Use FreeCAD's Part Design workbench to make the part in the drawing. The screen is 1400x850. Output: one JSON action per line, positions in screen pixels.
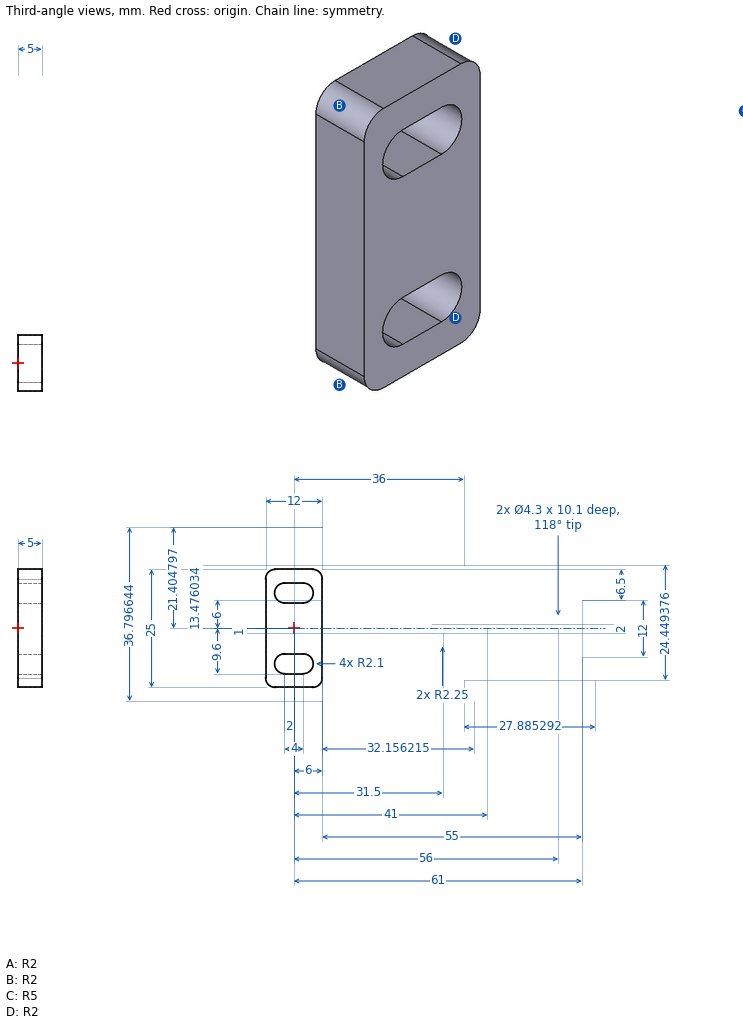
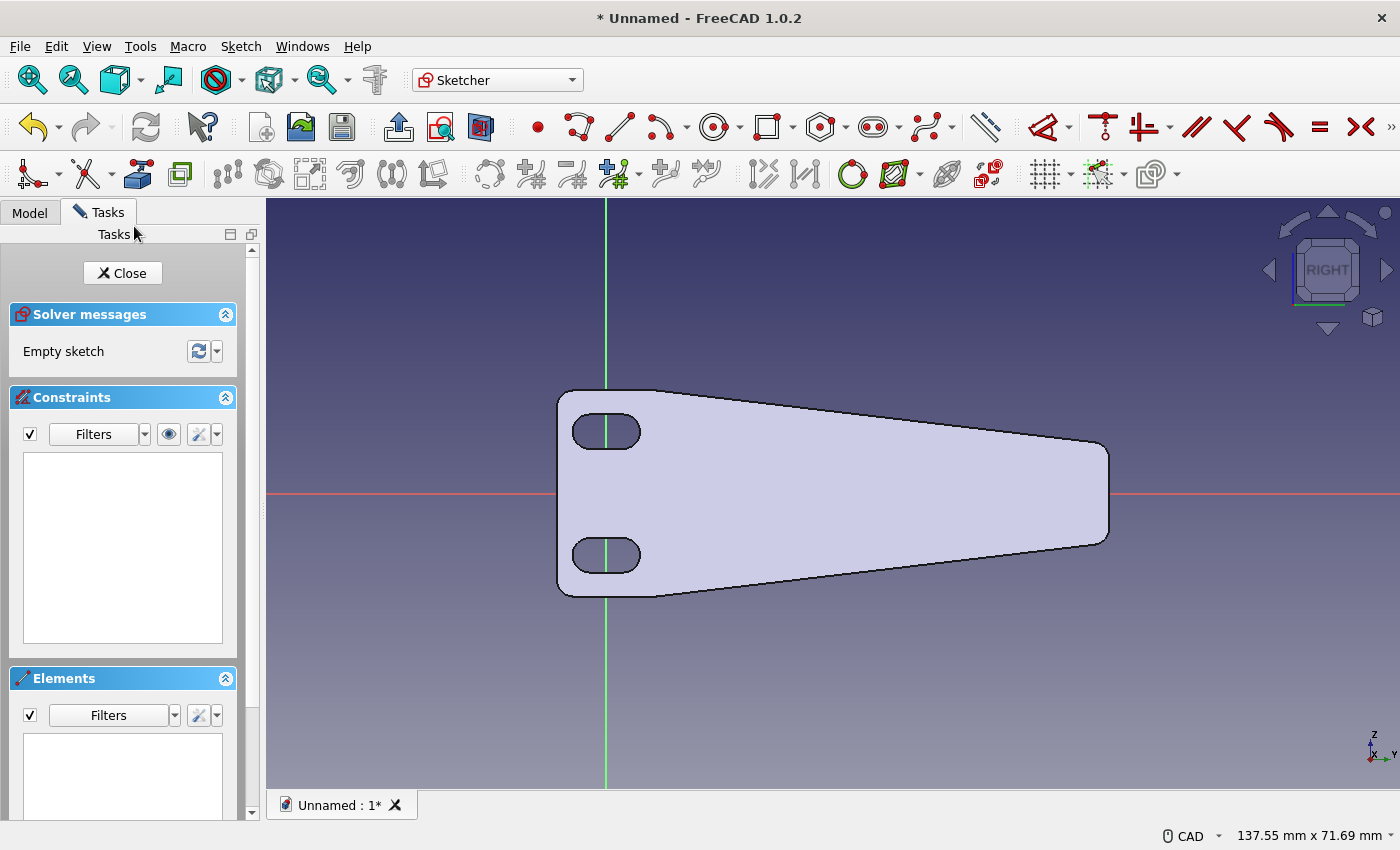
{"action": "left_click", "coordinate": [481, 128]}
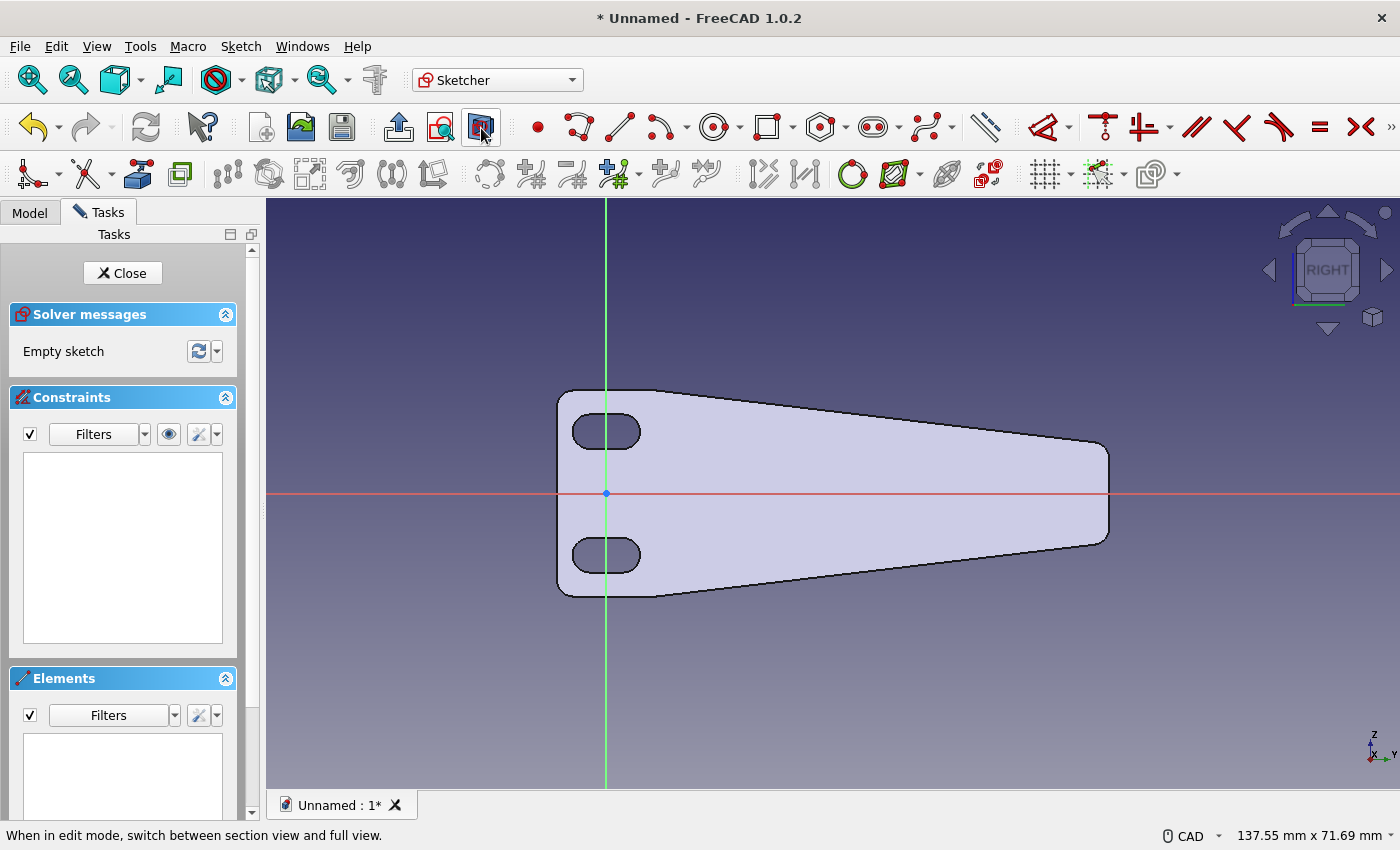
{"action": "scroll", "coordinate": [1085, 494], "scroll_direction": "up", "scroll_amount": 7}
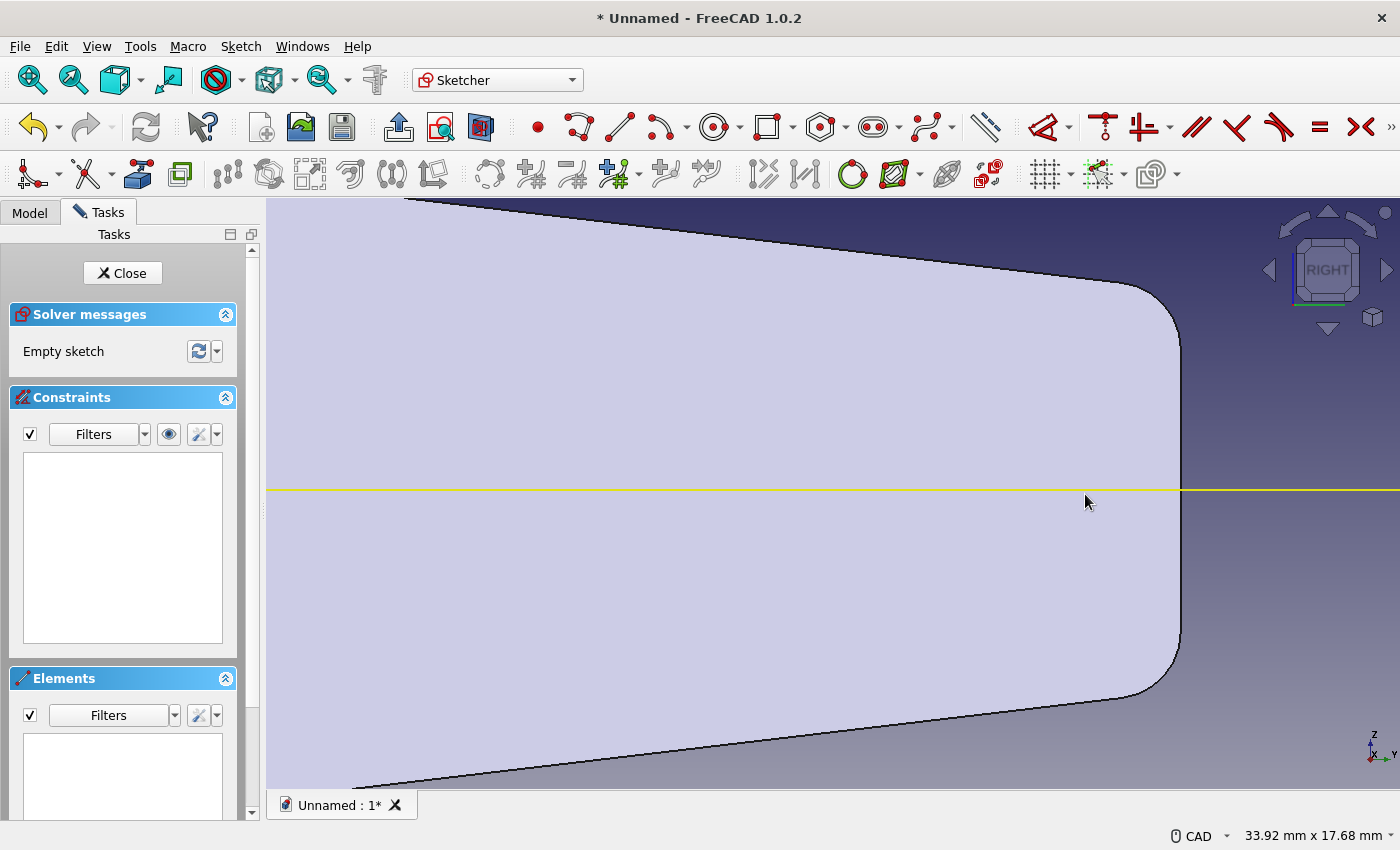
{"action": "left_click", "coordinate": [714, 128]}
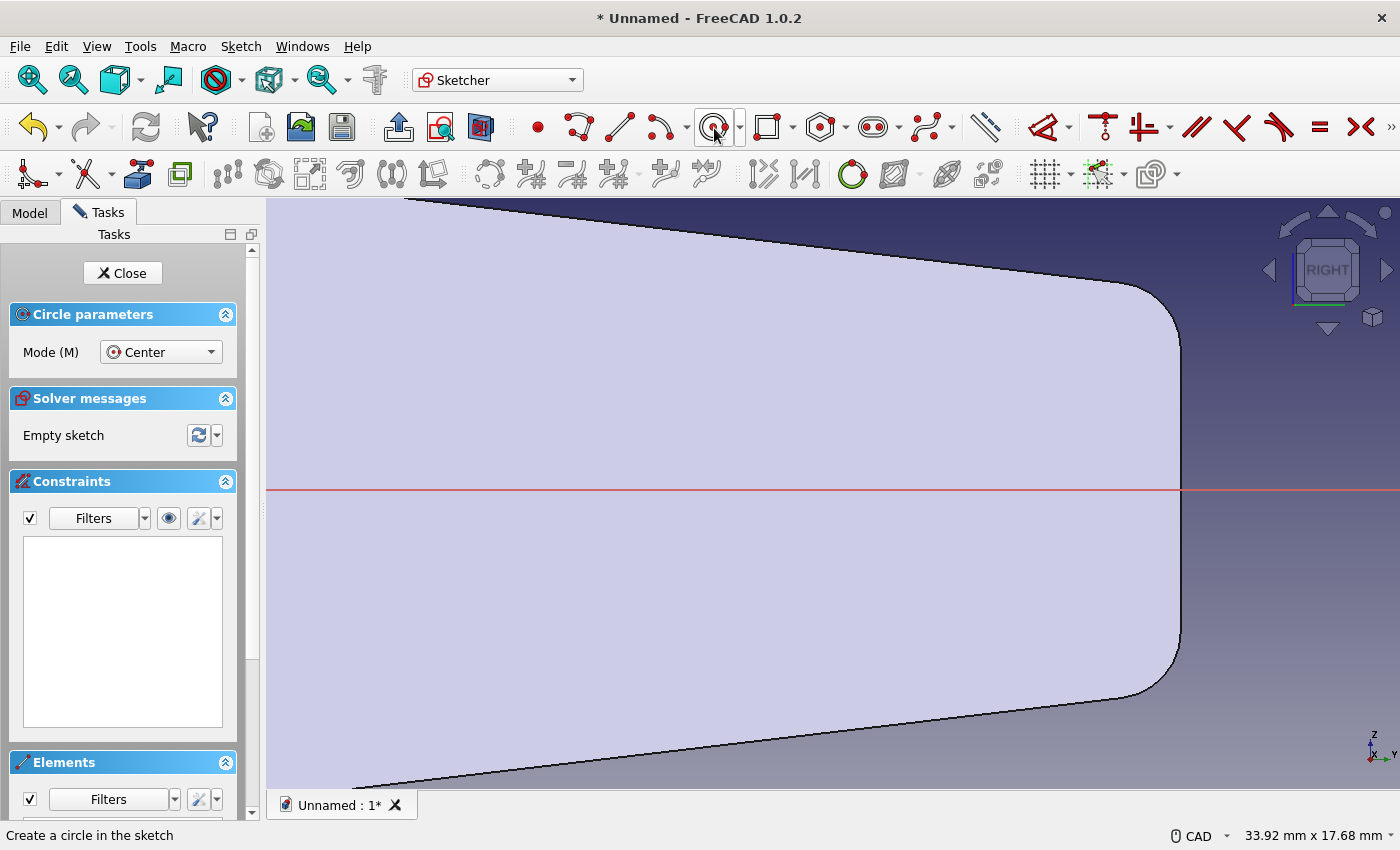
{"action": "left_click", "coordinate": [1014, 490]}
{"action": "left_click", "coordinate": [1065, 440]}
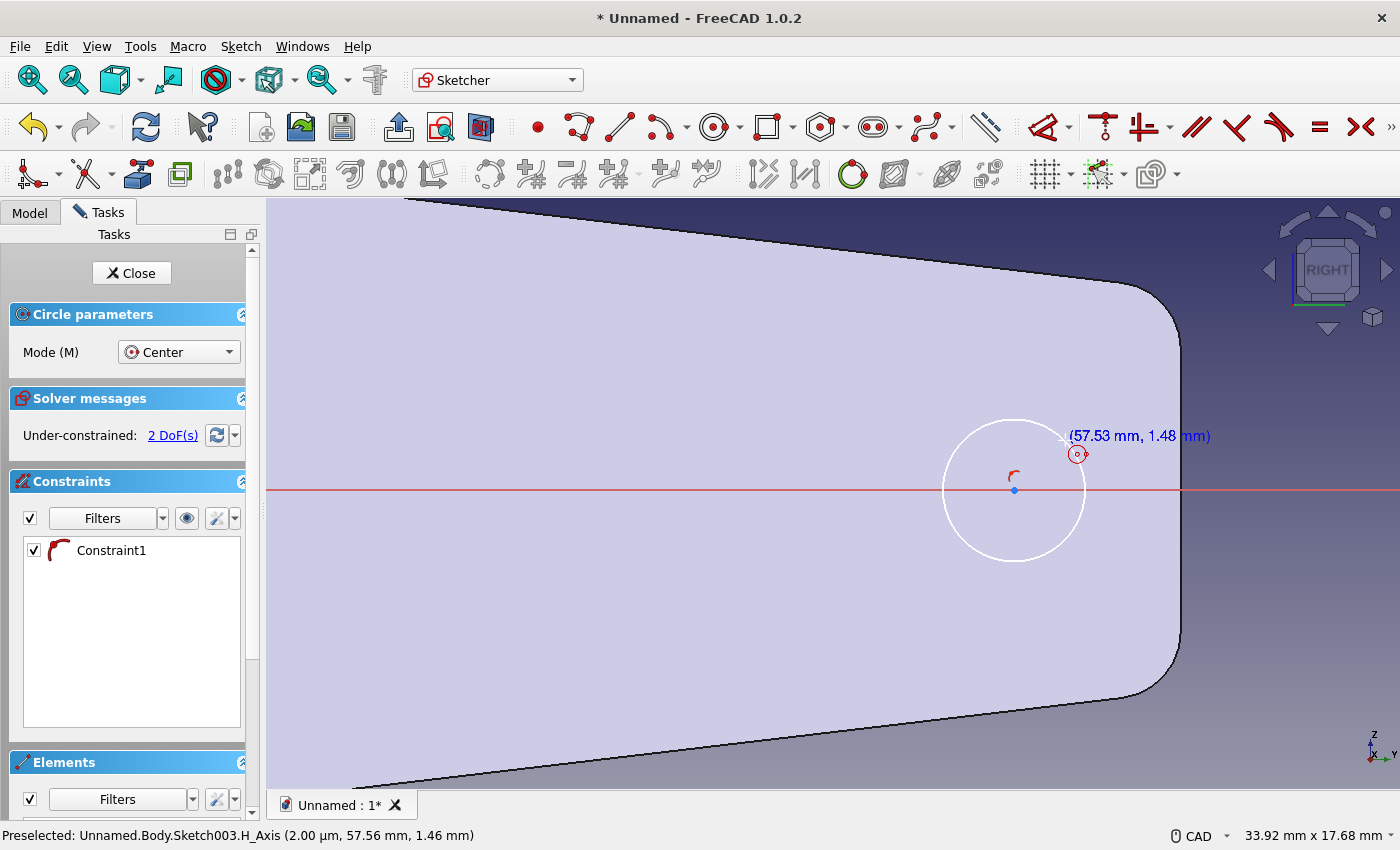
{"action": "left_click", "coordinate": [512, 490]}
{"action": "left_click", "coordinate": [563, 440]}
{"action": "key", "text": "Escape"}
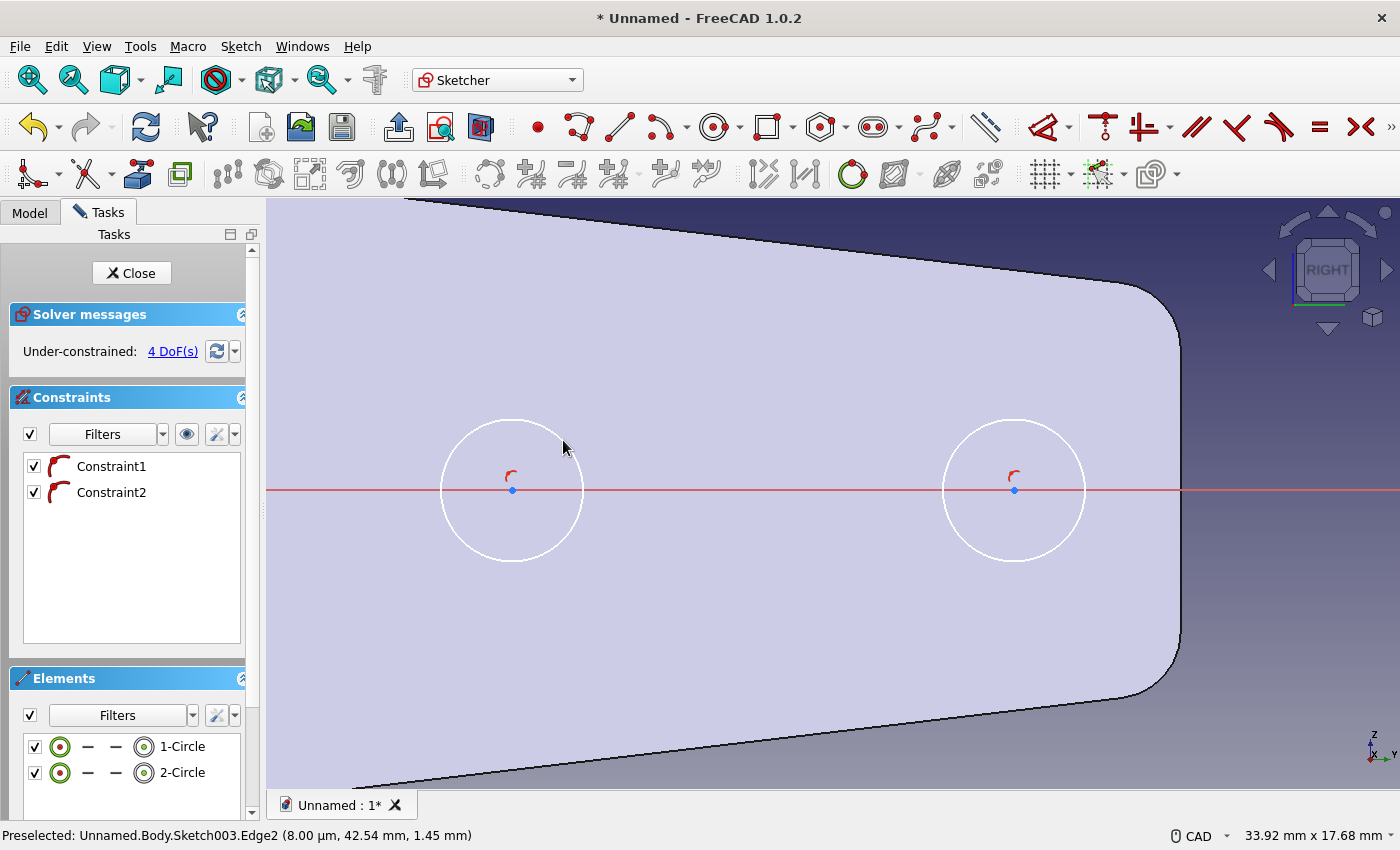
{"action": "left_click", "coordinate": [1064, 440]}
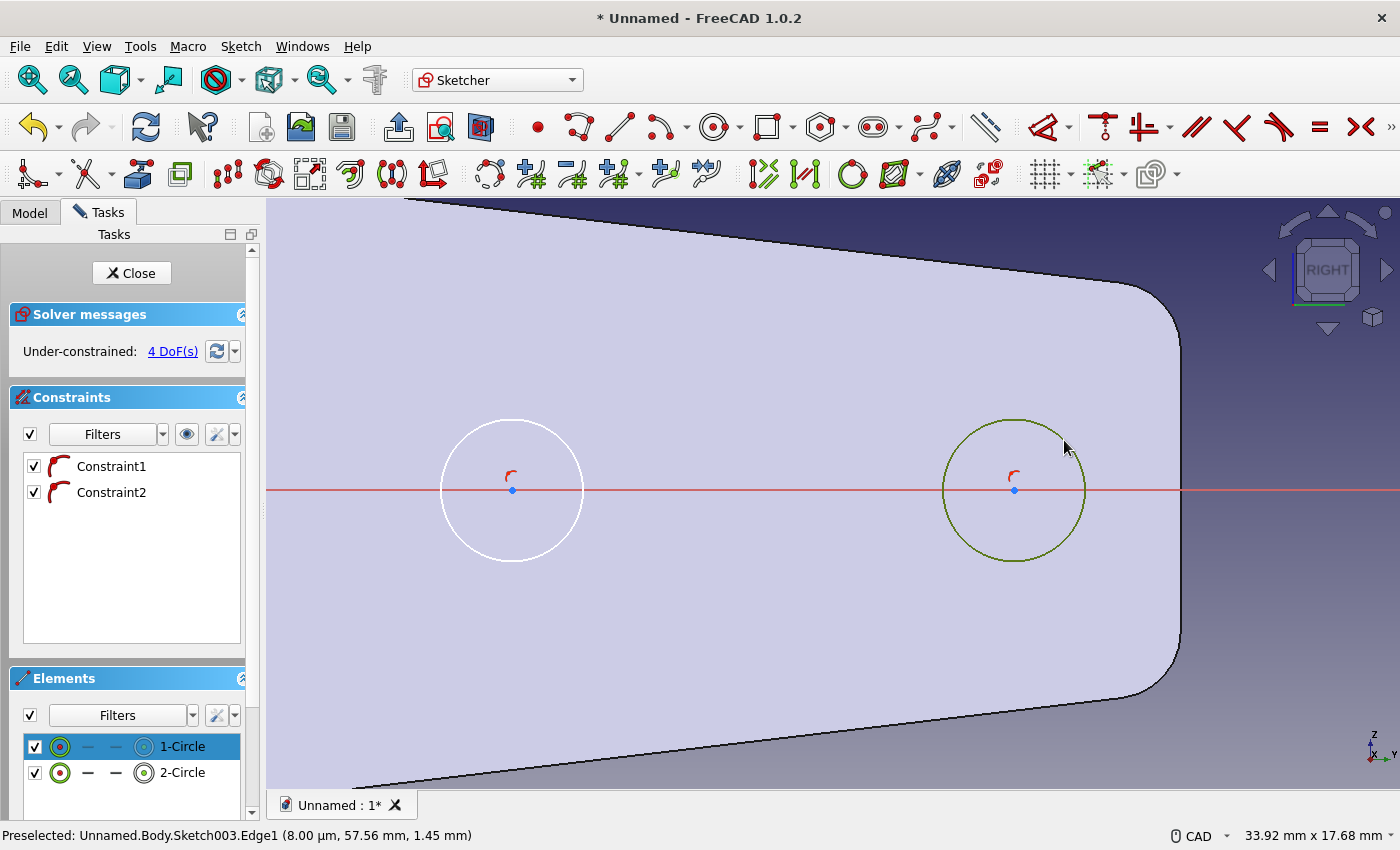
{"action": "left_click", "coordinate": [562, 440]}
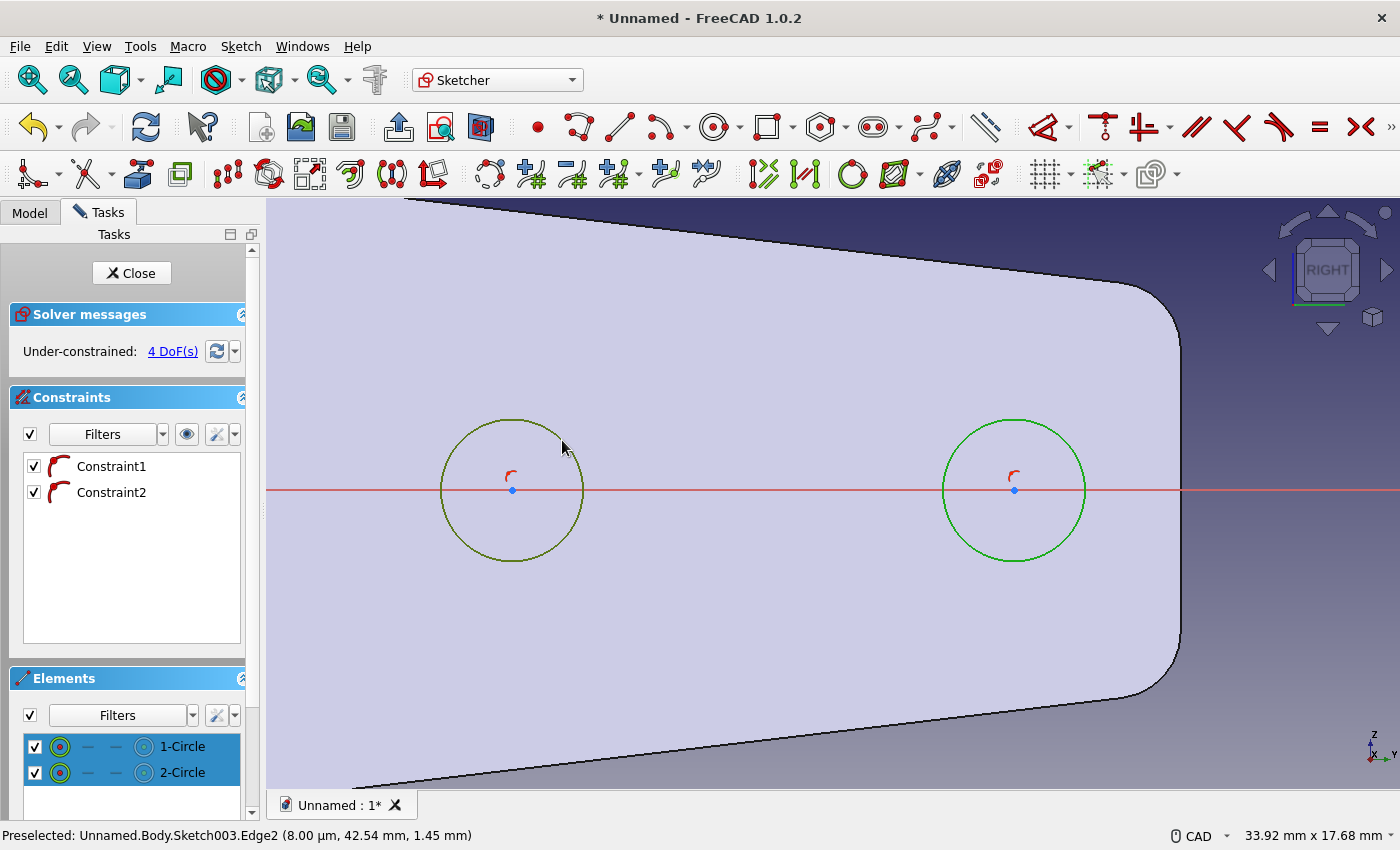
{"action": "key", "text": "e"}